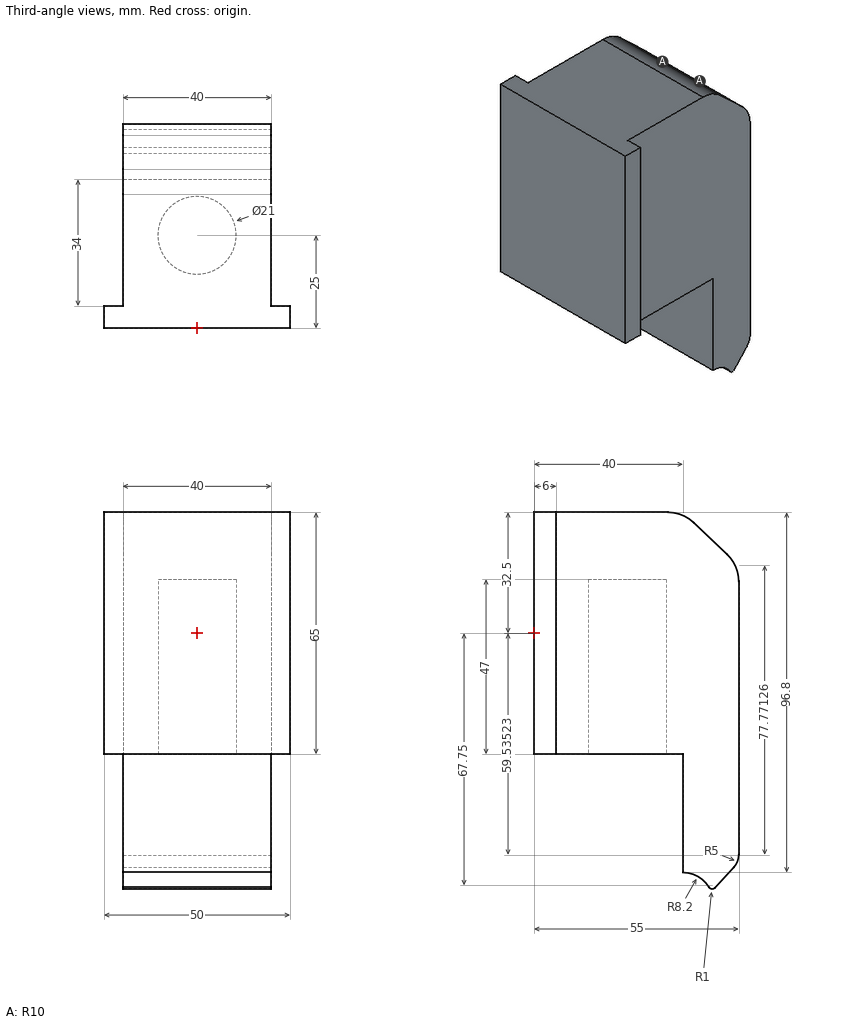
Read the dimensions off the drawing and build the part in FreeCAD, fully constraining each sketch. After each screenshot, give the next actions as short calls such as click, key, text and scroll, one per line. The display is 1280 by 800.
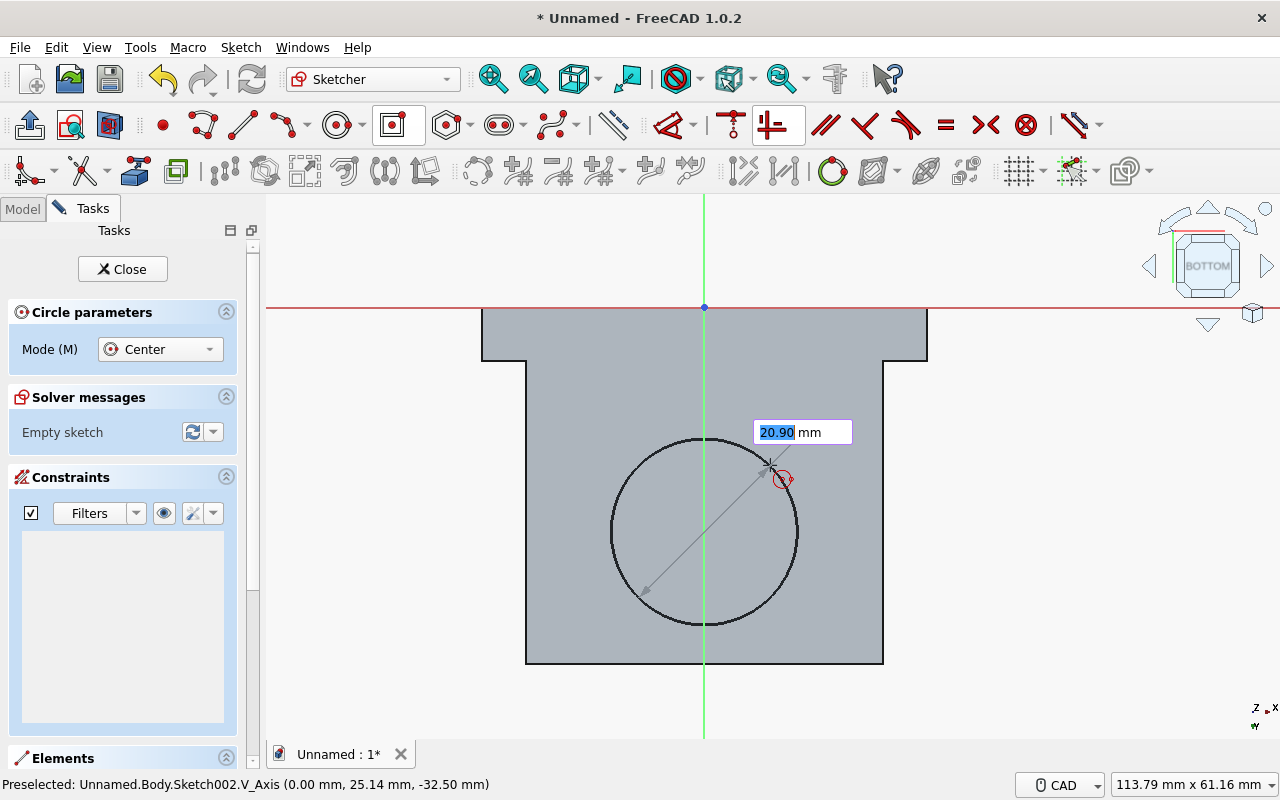
text(21)
key(Return)
key(Escape)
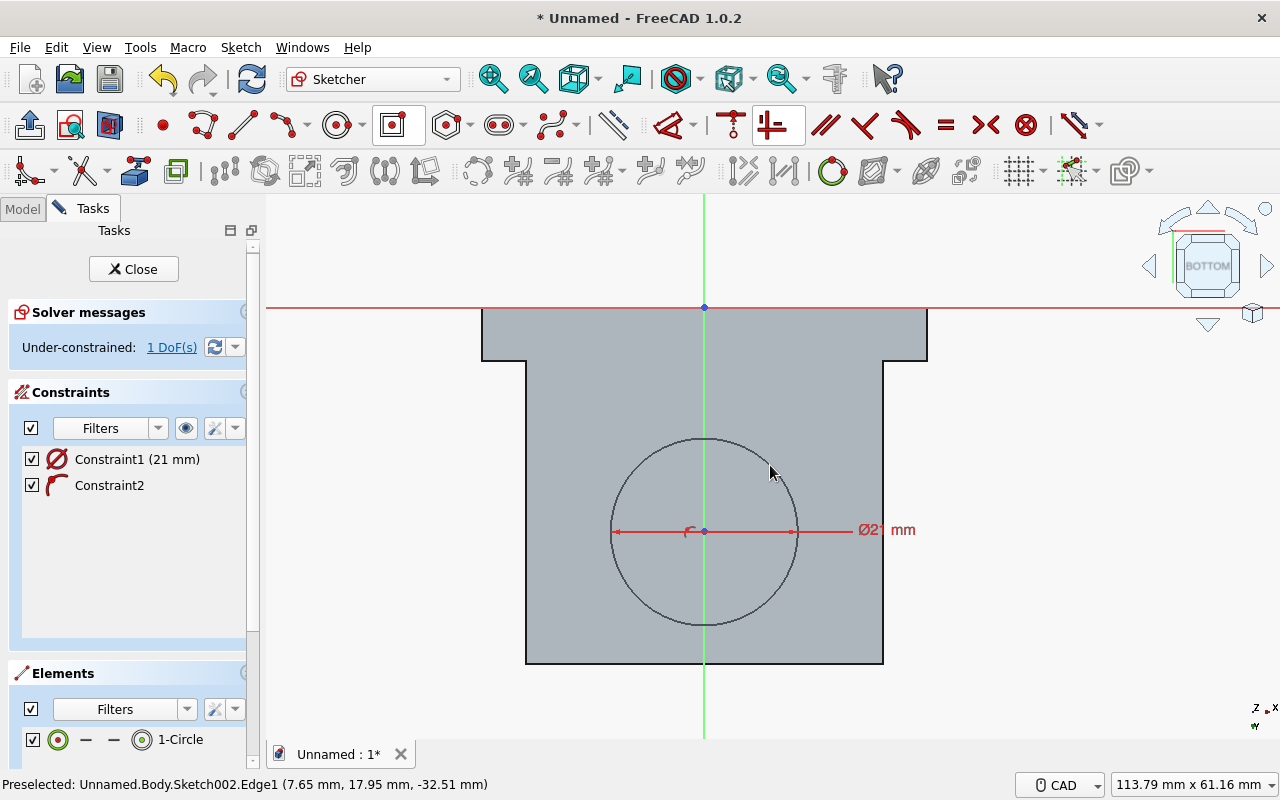
click(668, 126)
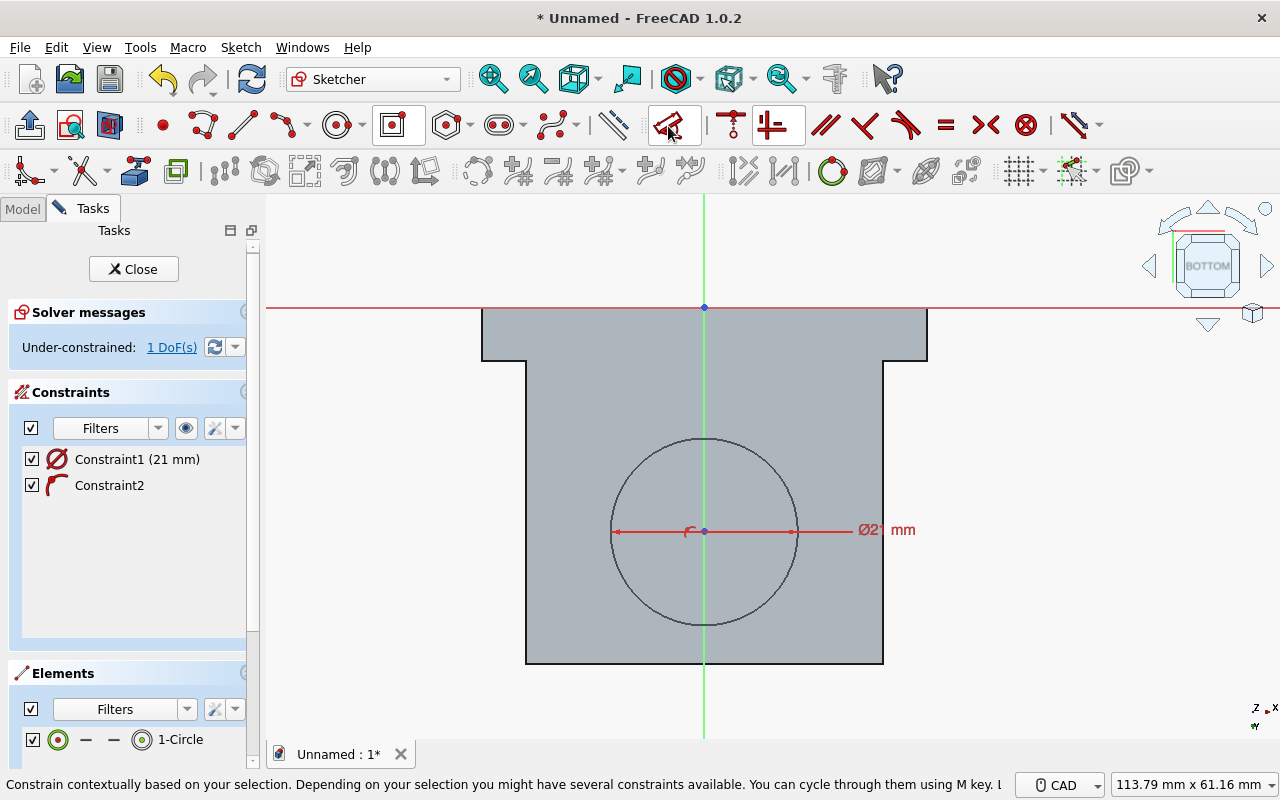
click(704, 532)
click(738, 420)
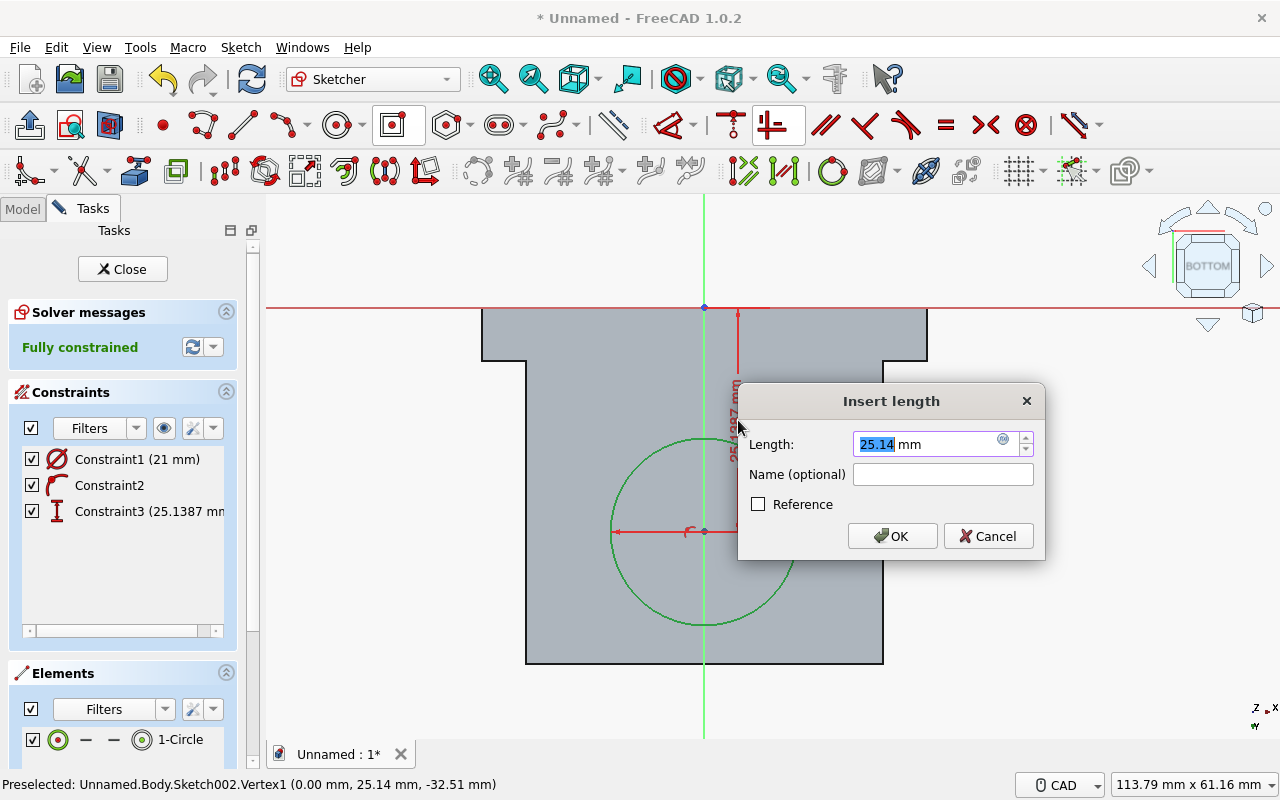
text(25)
key(Return)
key(Escape)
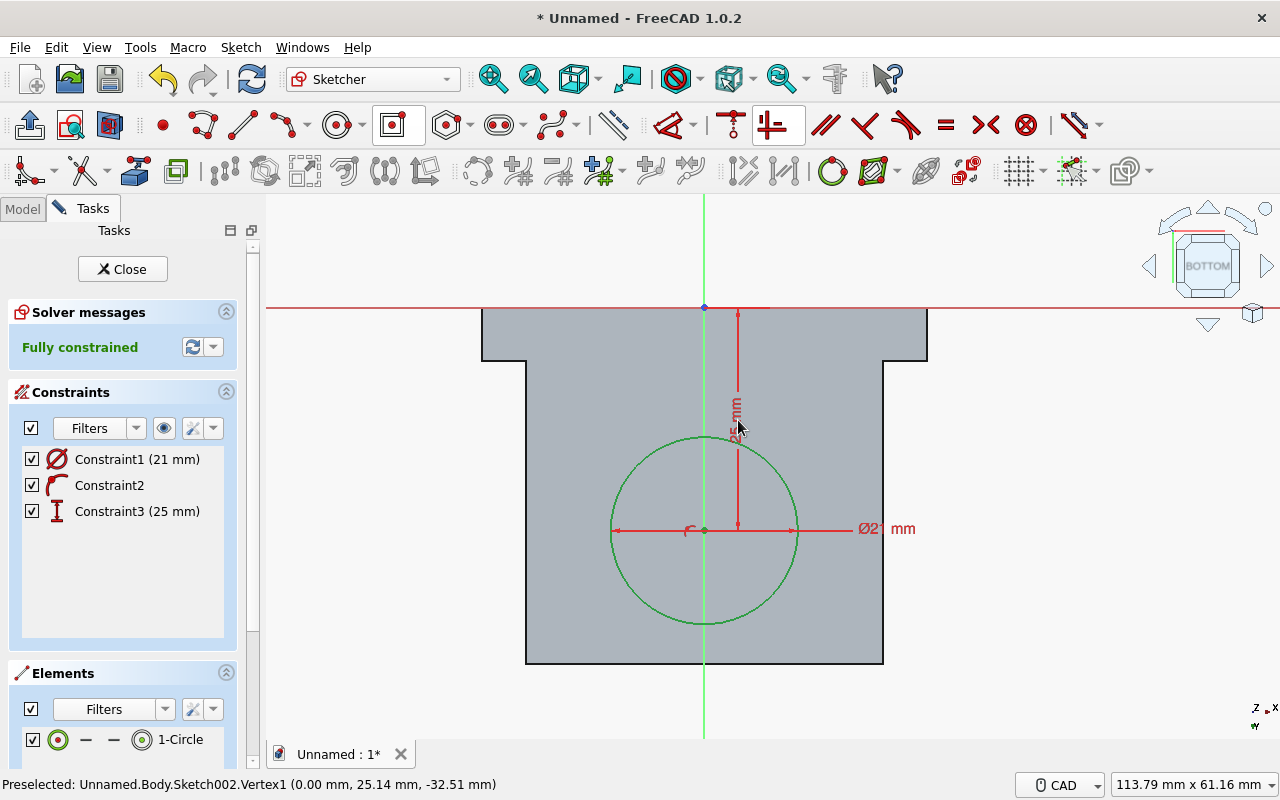
click(123, 269)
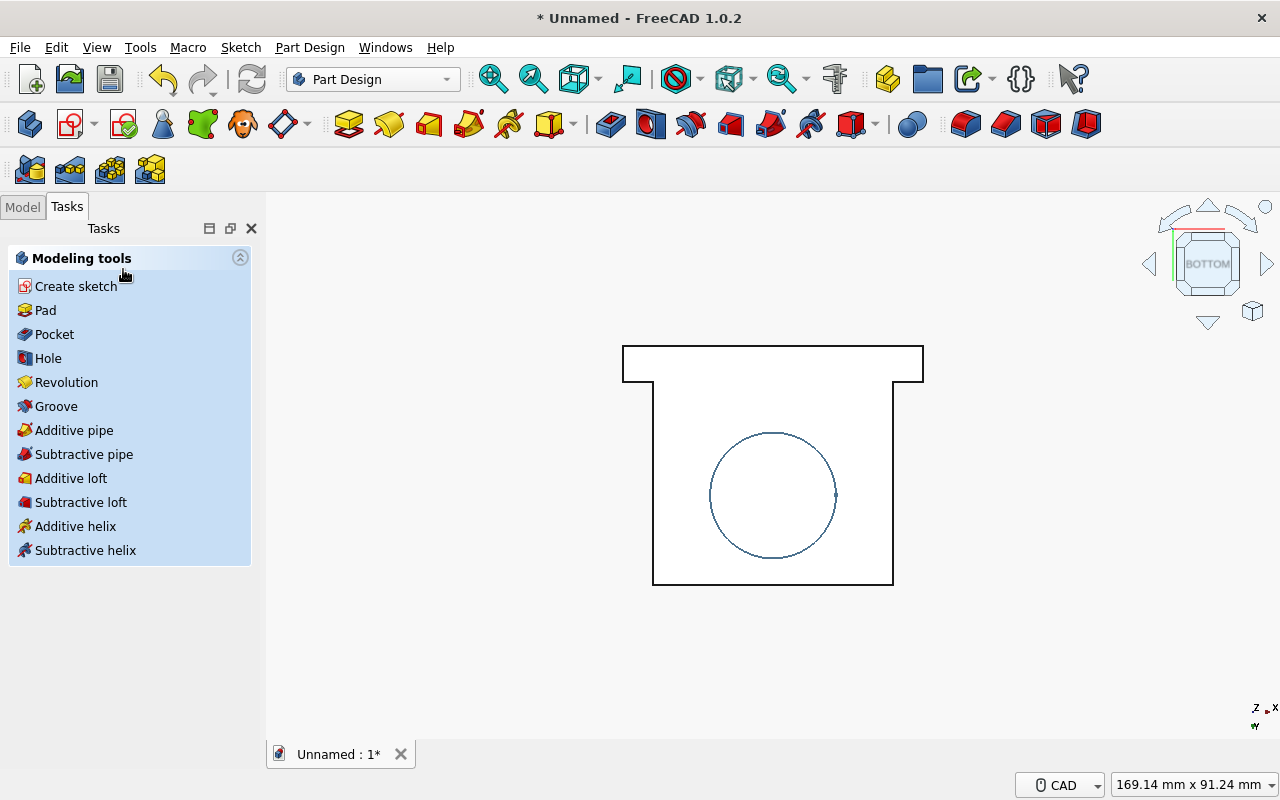
click(612, 124)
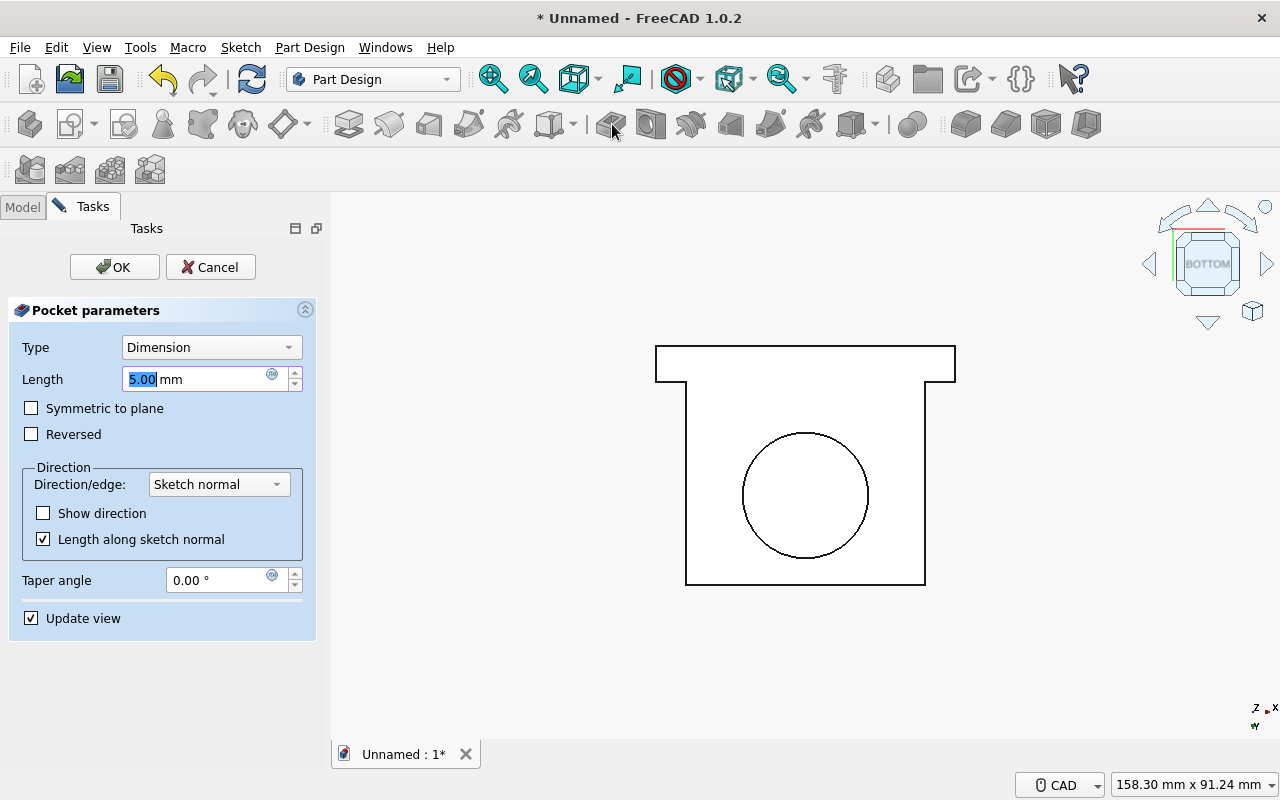
text(47)
key(Tab)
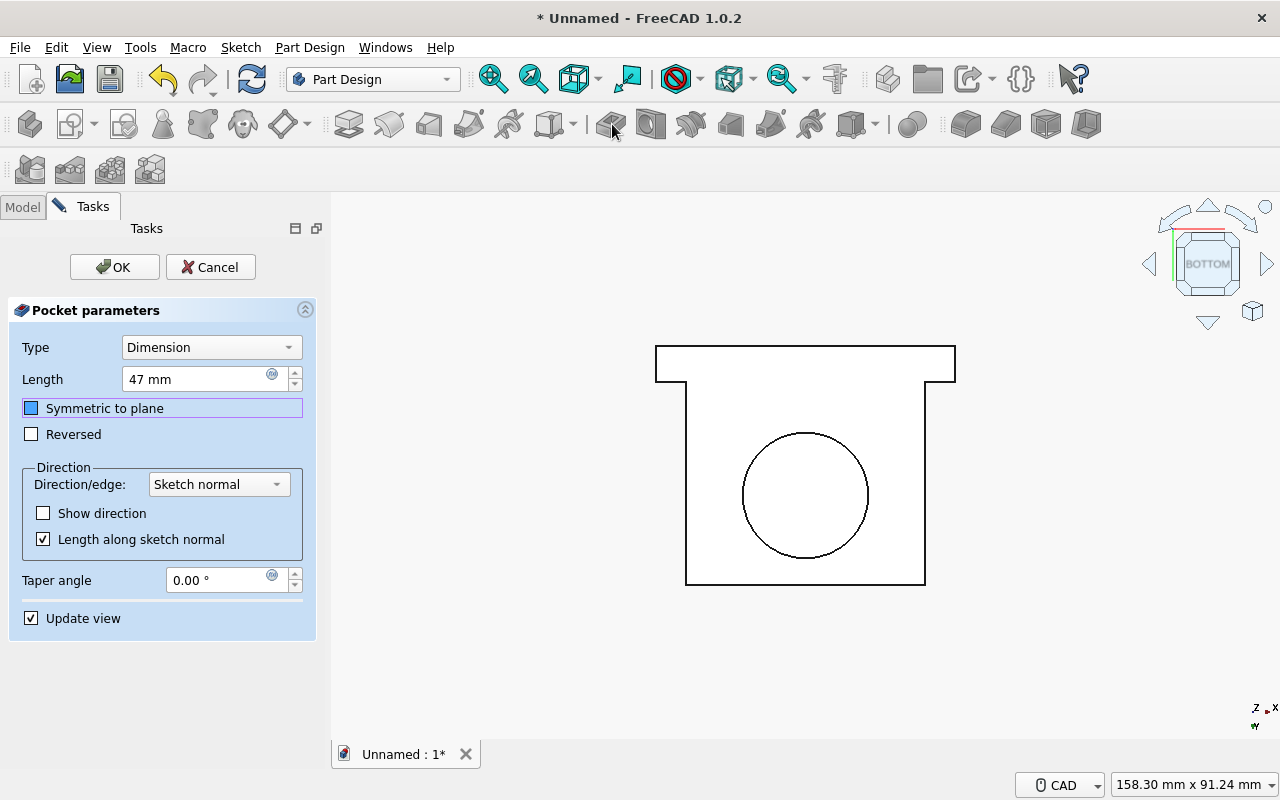
click(115, 267)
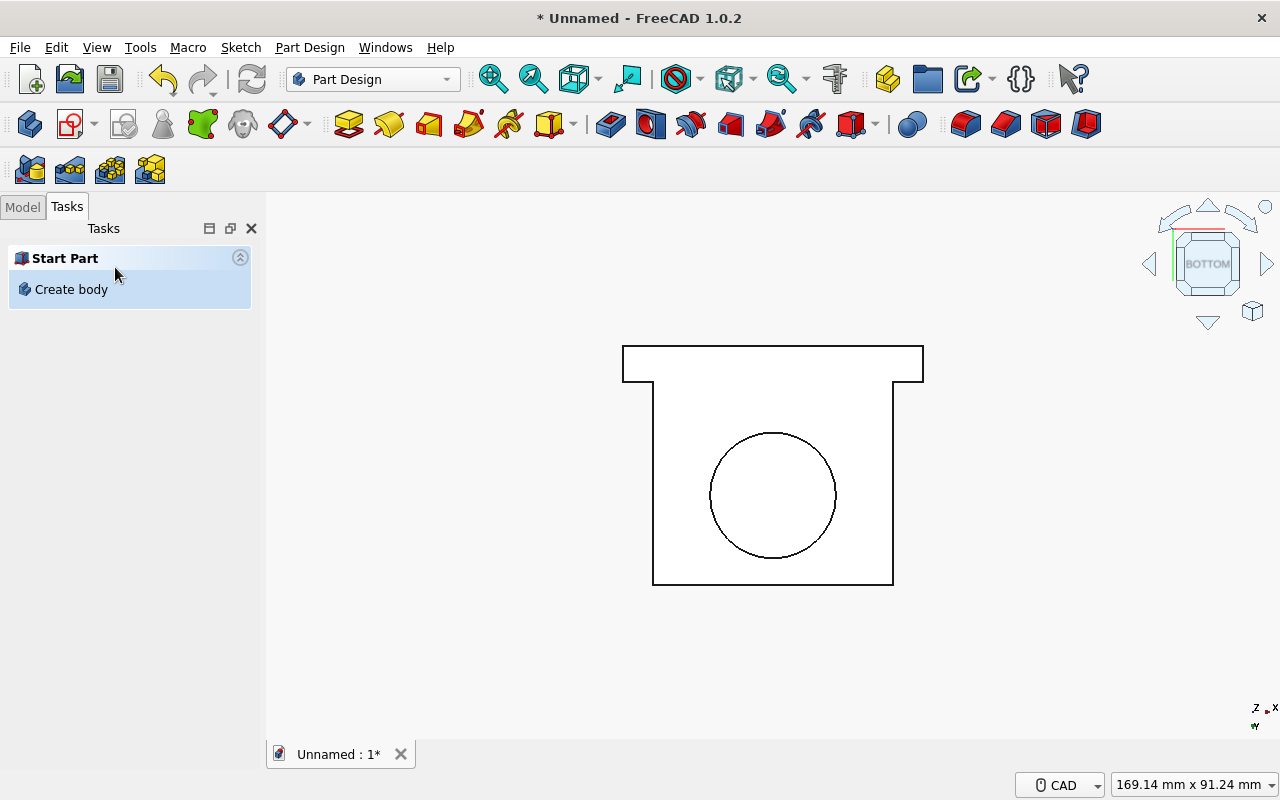
key(v)
key(f)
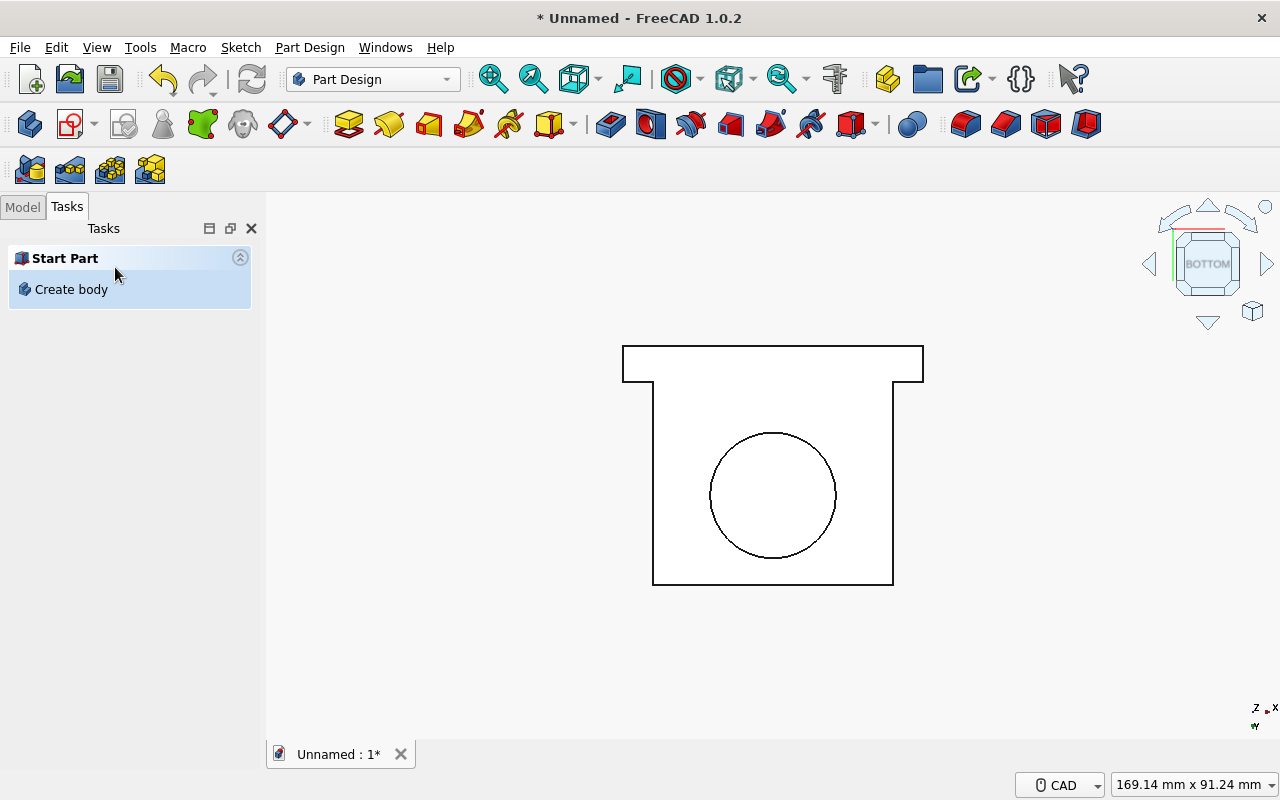
click(70, 124)